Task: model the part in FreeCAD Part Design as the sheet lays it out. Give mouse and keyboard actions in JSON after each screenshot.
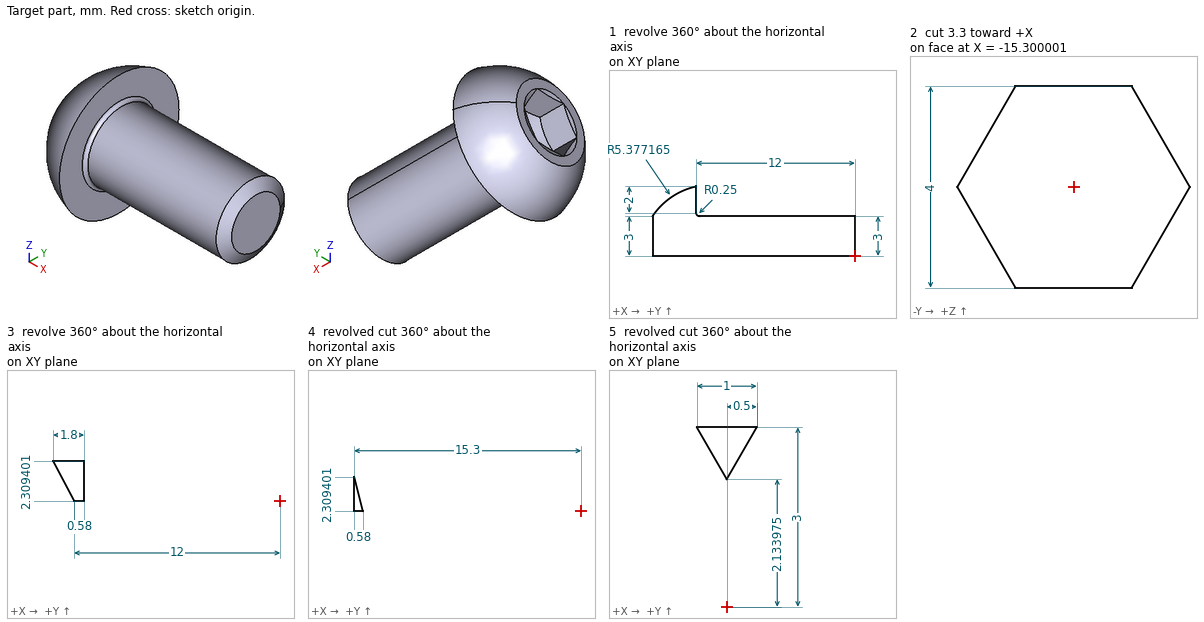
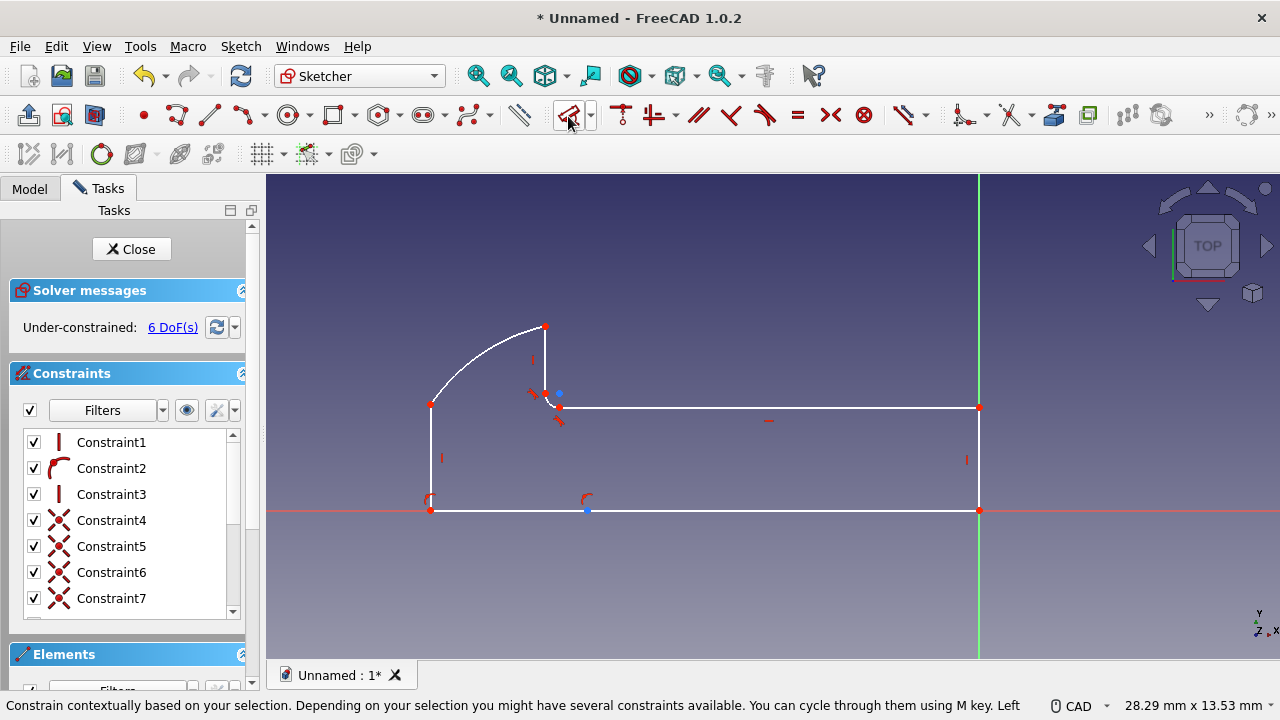
{"action": "left_click", "coordinate": [505, 340]}
{"action": "left_click", "coordinate": [491, 311]}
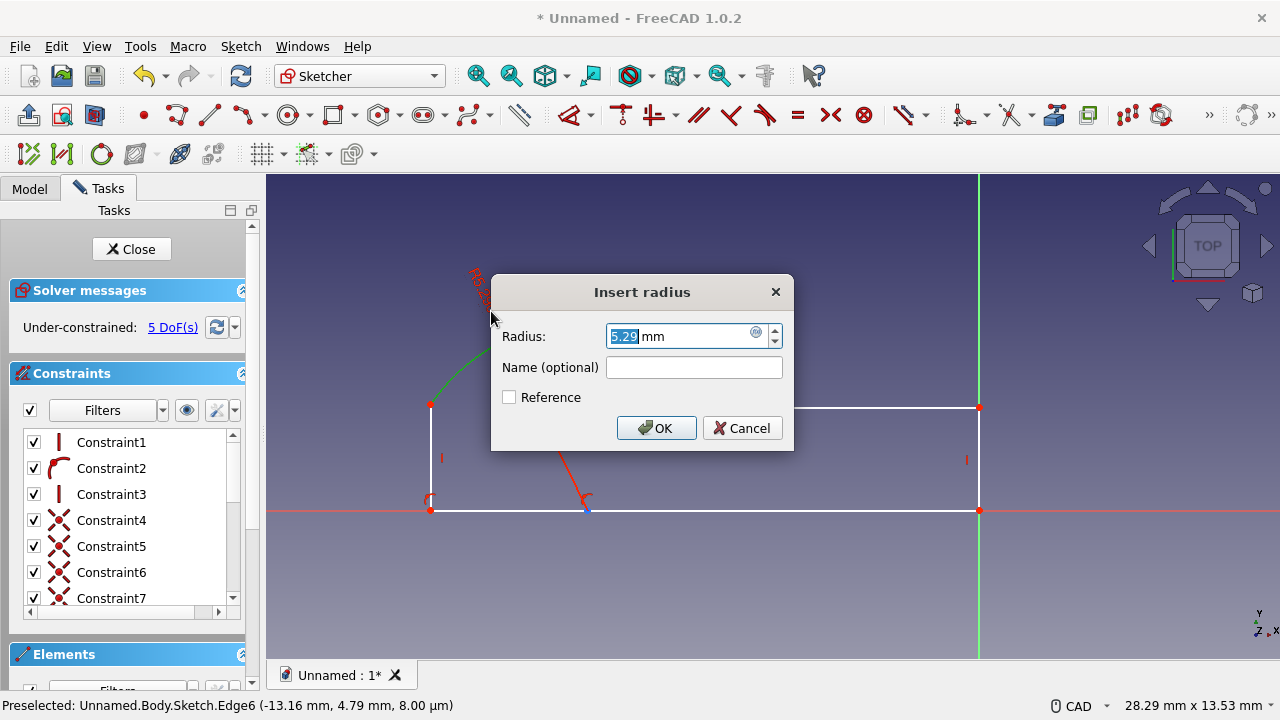
{"action": "type", "text": "5.377165"}
{"action": "key", "text": "Return"}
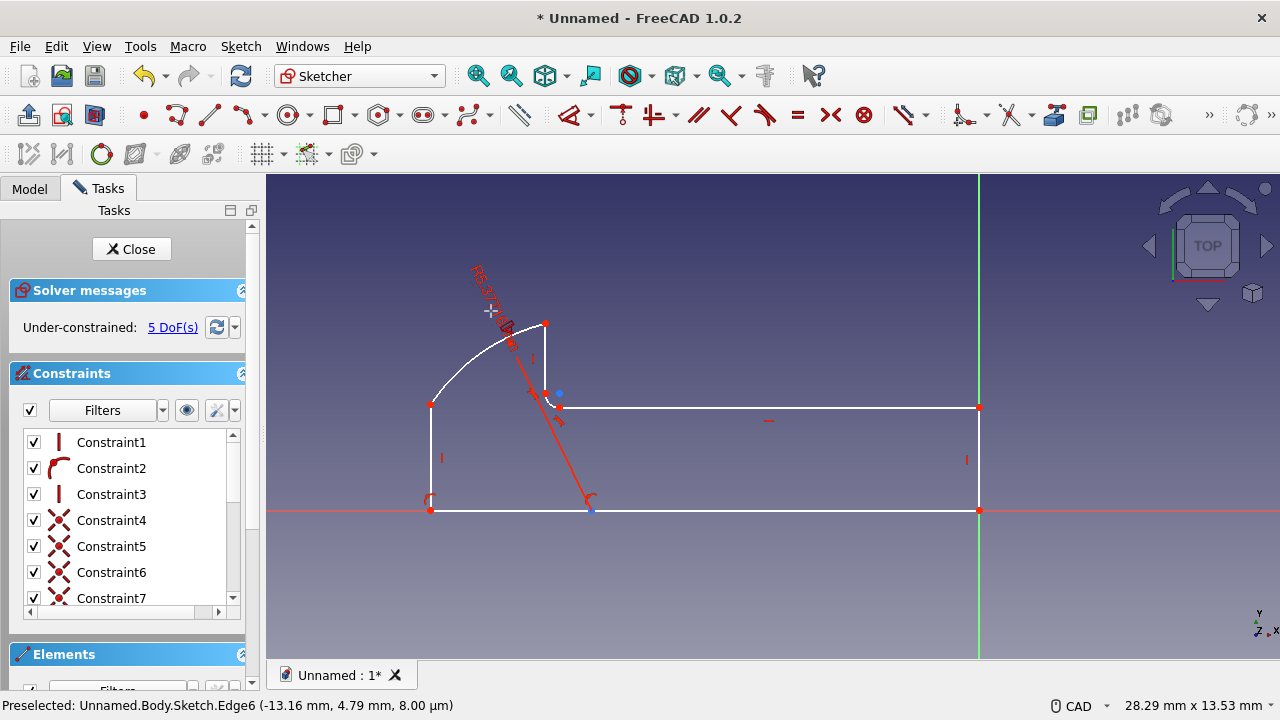
{"action": "scroll", "coordinate": [550, 404], "scroll_direction": "up", "scroll_amount": 8}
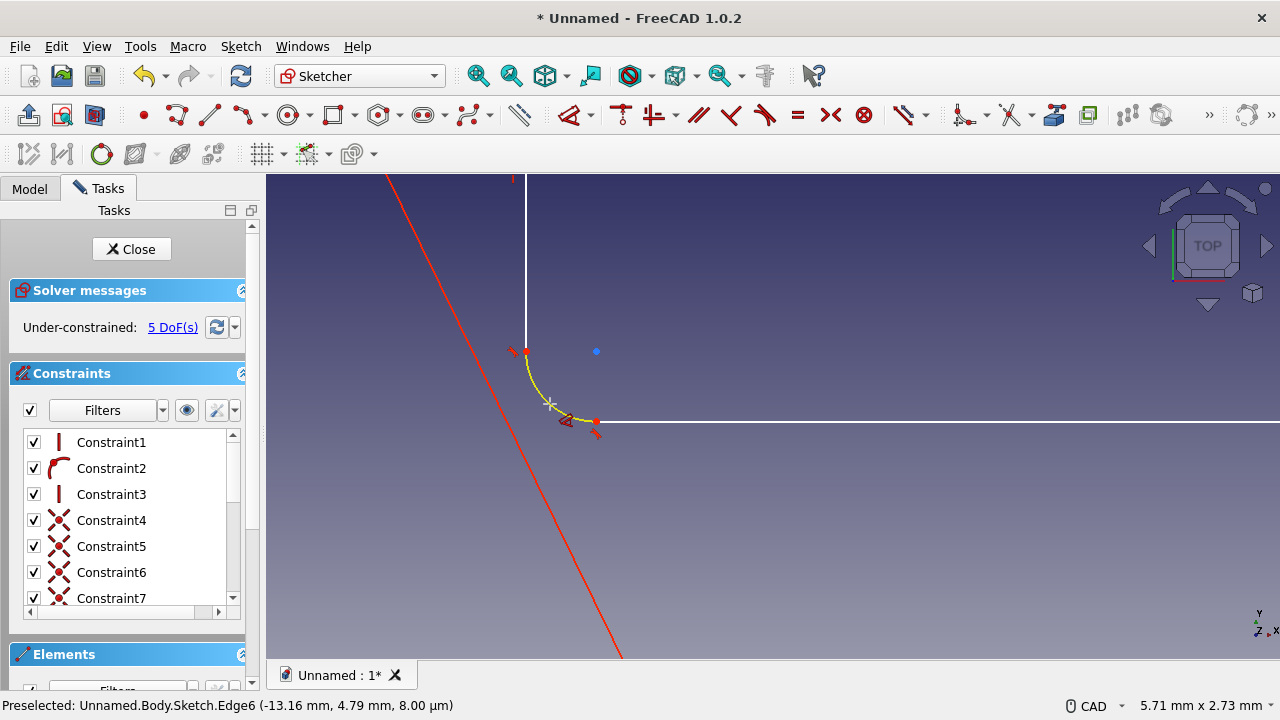
{"action": "left_click", "coordinate": [547, 401]}
{"action": "left_click", "coordinate": [524, 424]}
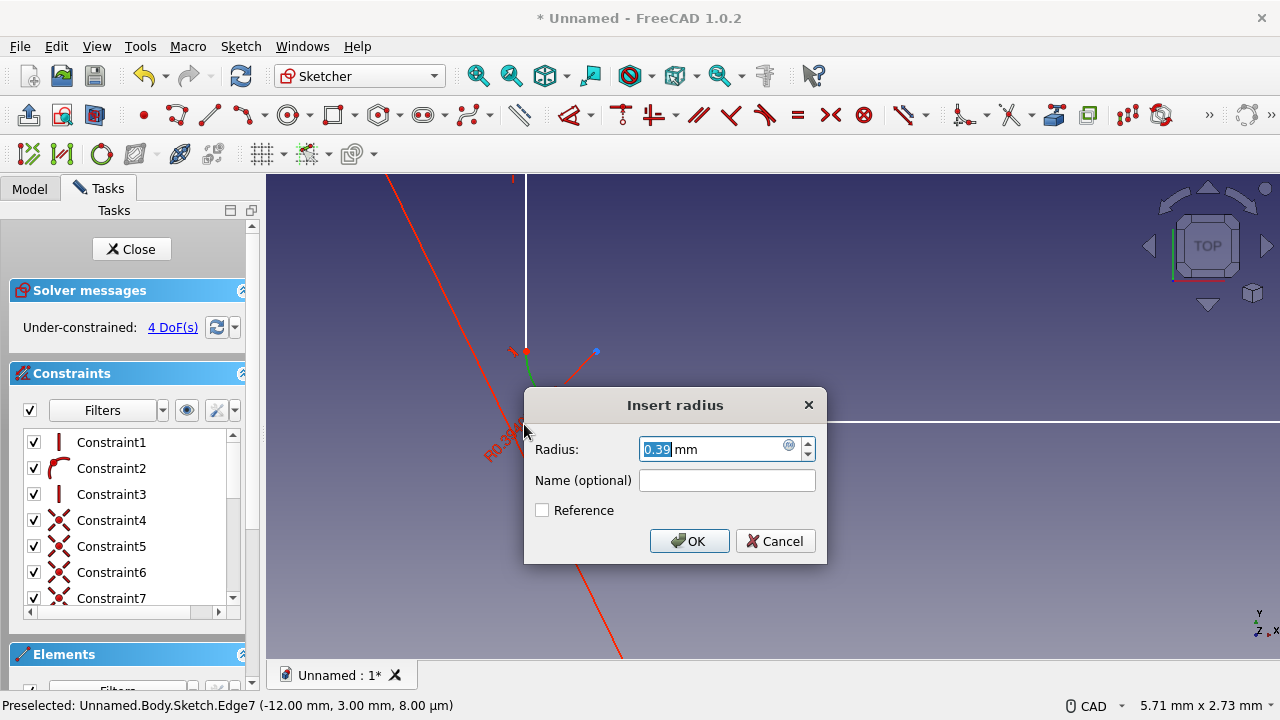
{"action": "type", "text": "0.25"}
{"action": "key", "text": "Return"}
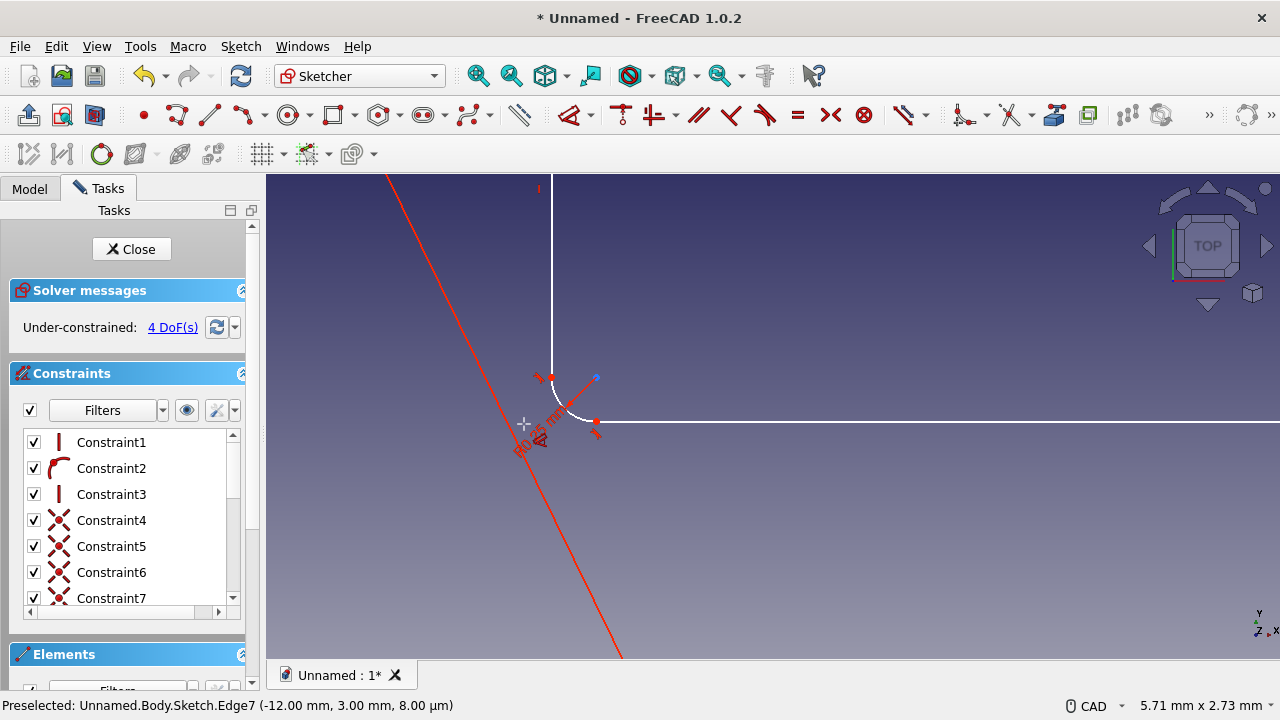
{"action": "scroll", "coordinate": [550, 404], "scroll_direction": "down", "scroll_amount": 8}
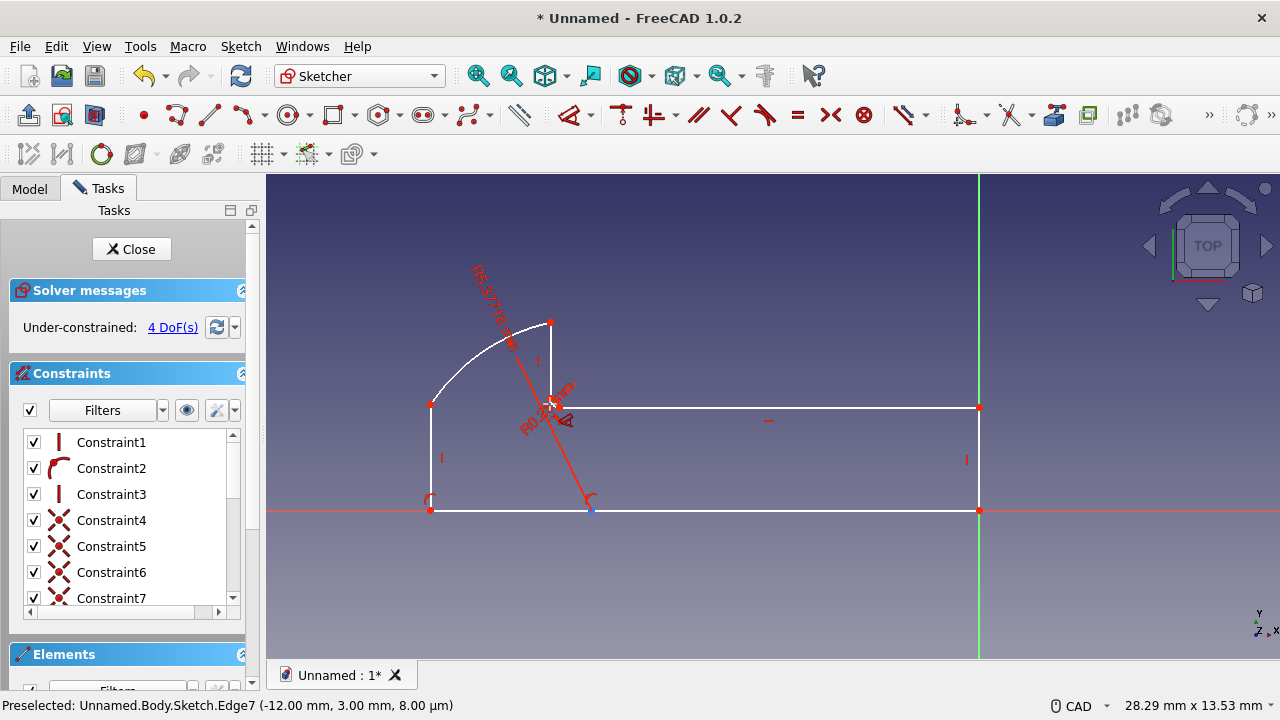
{"action": "left_click", "coordinate": [551, 376]}
{"action": "left_click", "coordinate": [517, 361]}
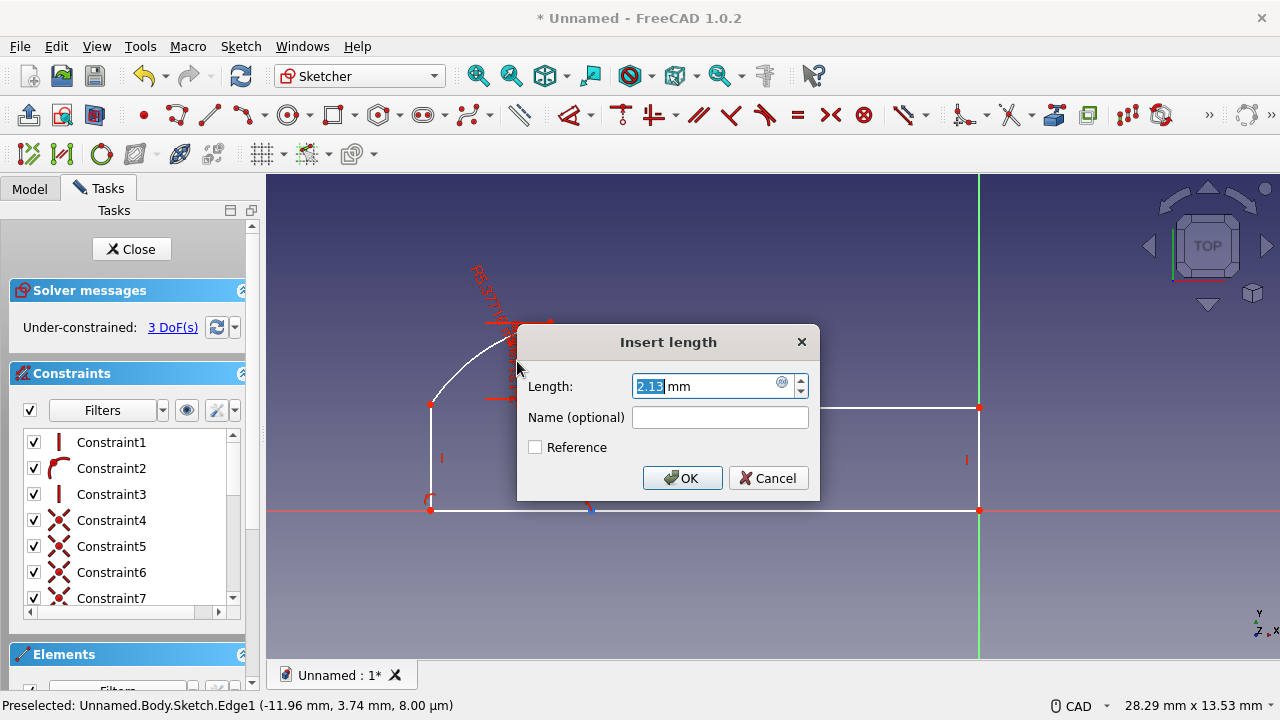
{"action": "type", "text": "2"}
{"action": "key", "text": "Return"}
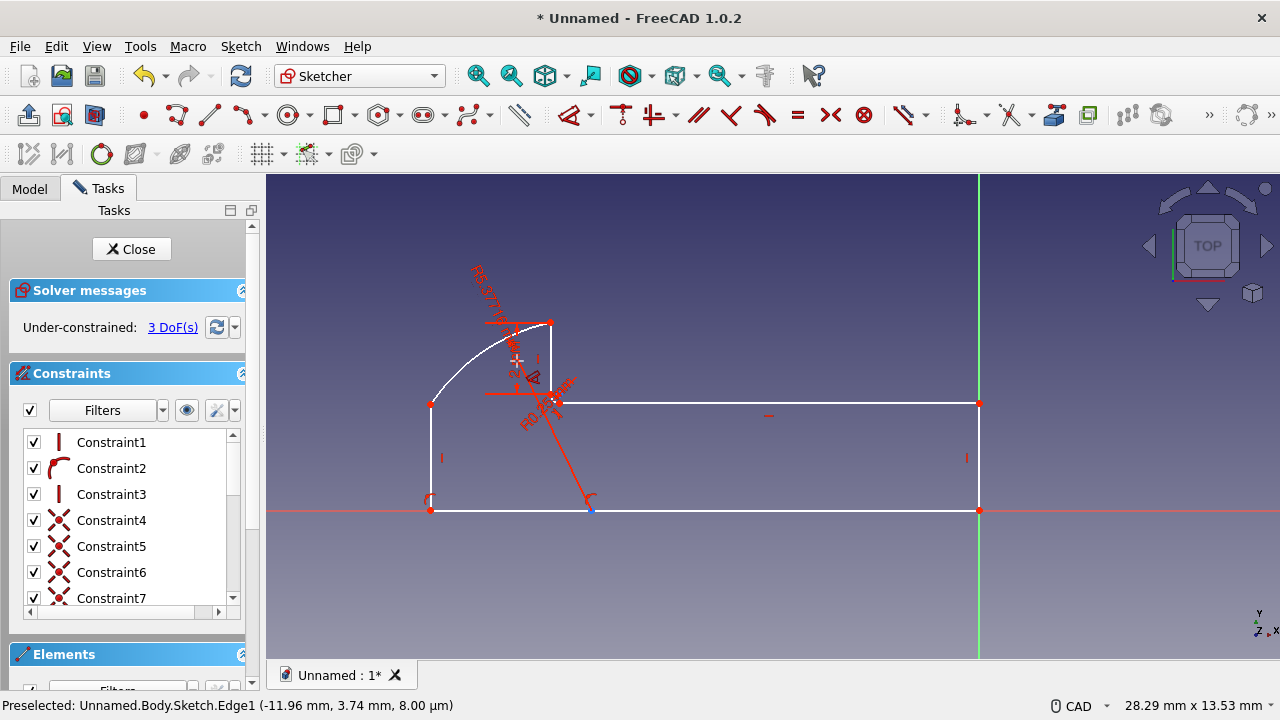
{"action": "left_click", "coordinate": [431, 437]}
{"action": "left_click", "coordinate": [397, 458]}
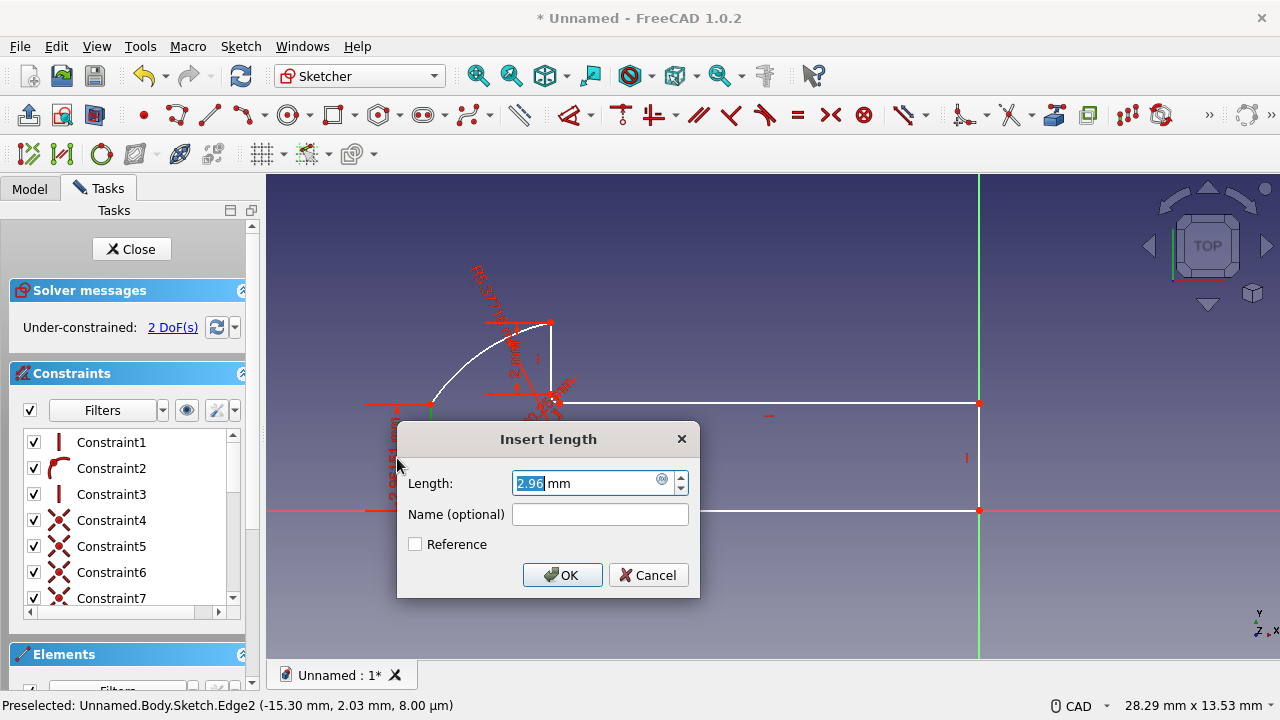
{"action": "type", "text": "3"}
{"action": "key", "text": "Return"}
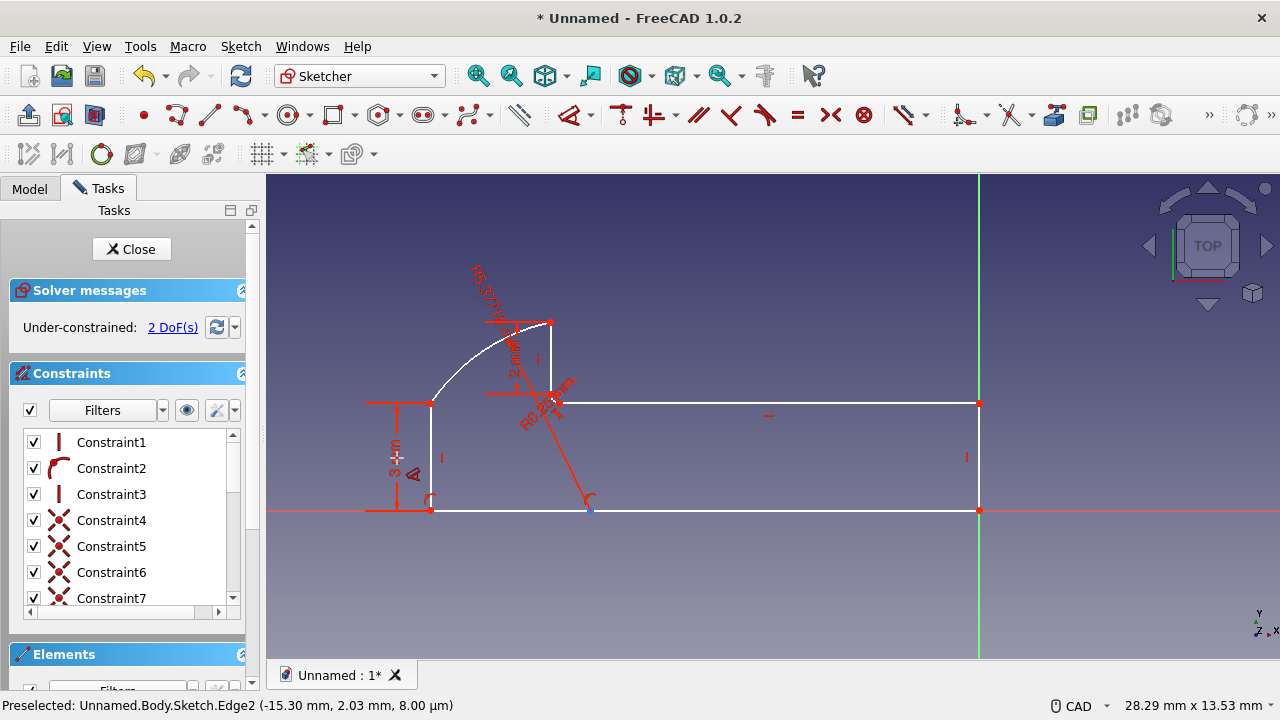
{"action": "left_click", "coordinate": [979, 403]}
{"action": "left_click", "coordinate": [1013, 457]}